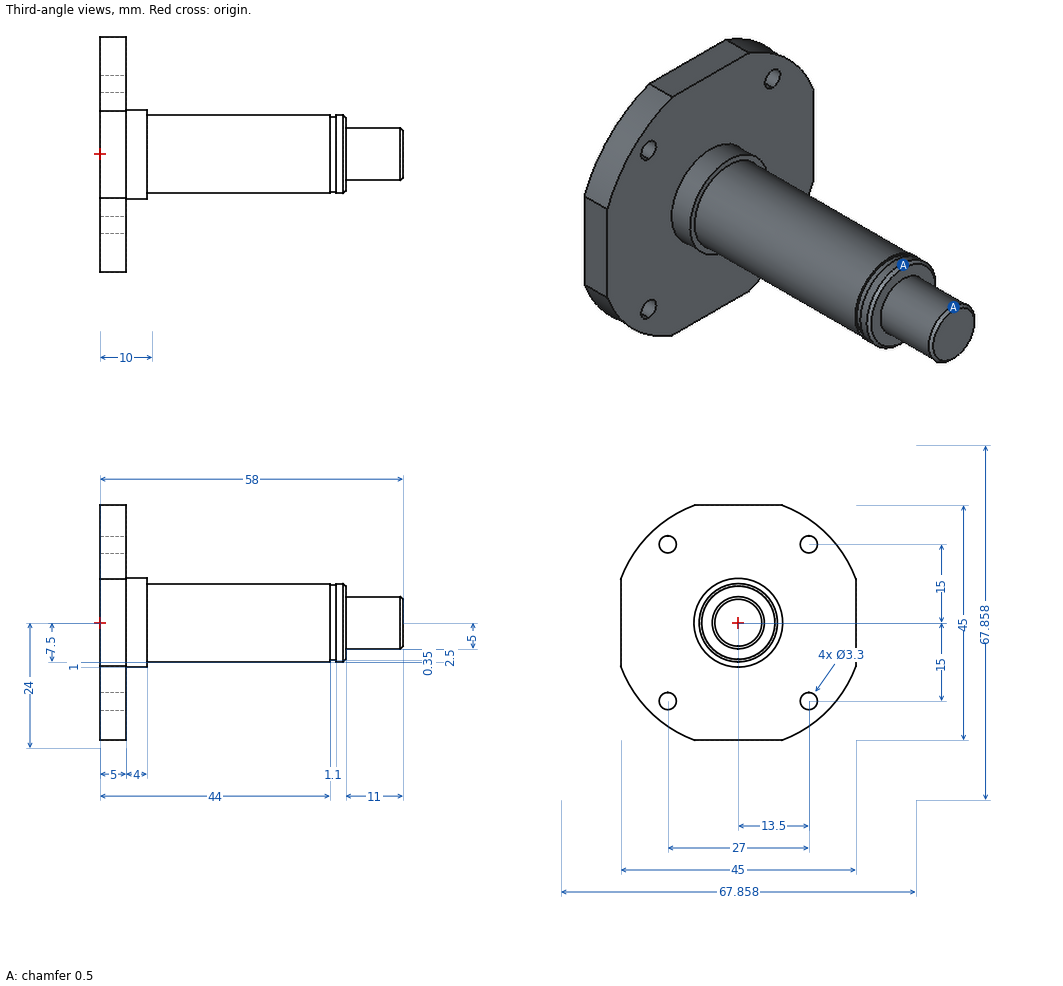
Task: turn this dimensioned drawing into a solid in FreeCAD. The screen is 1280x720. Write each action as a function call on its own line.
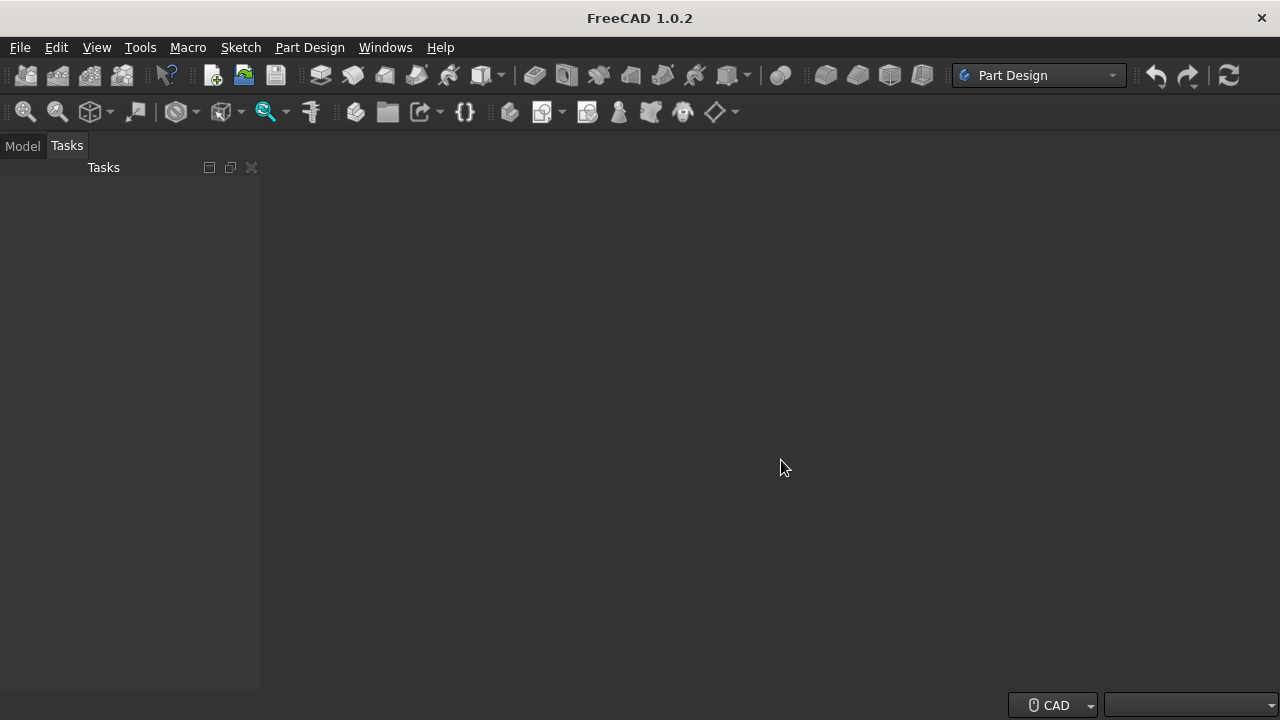
click(212, 76)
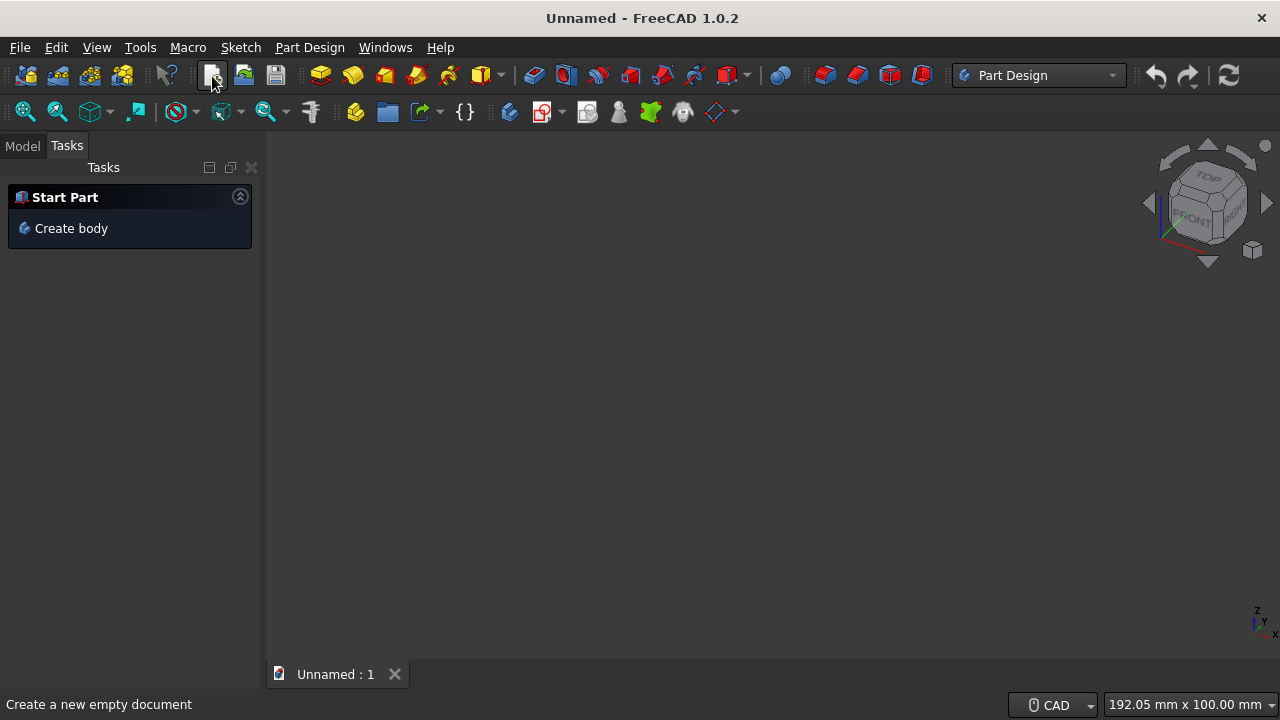
click(542, 112)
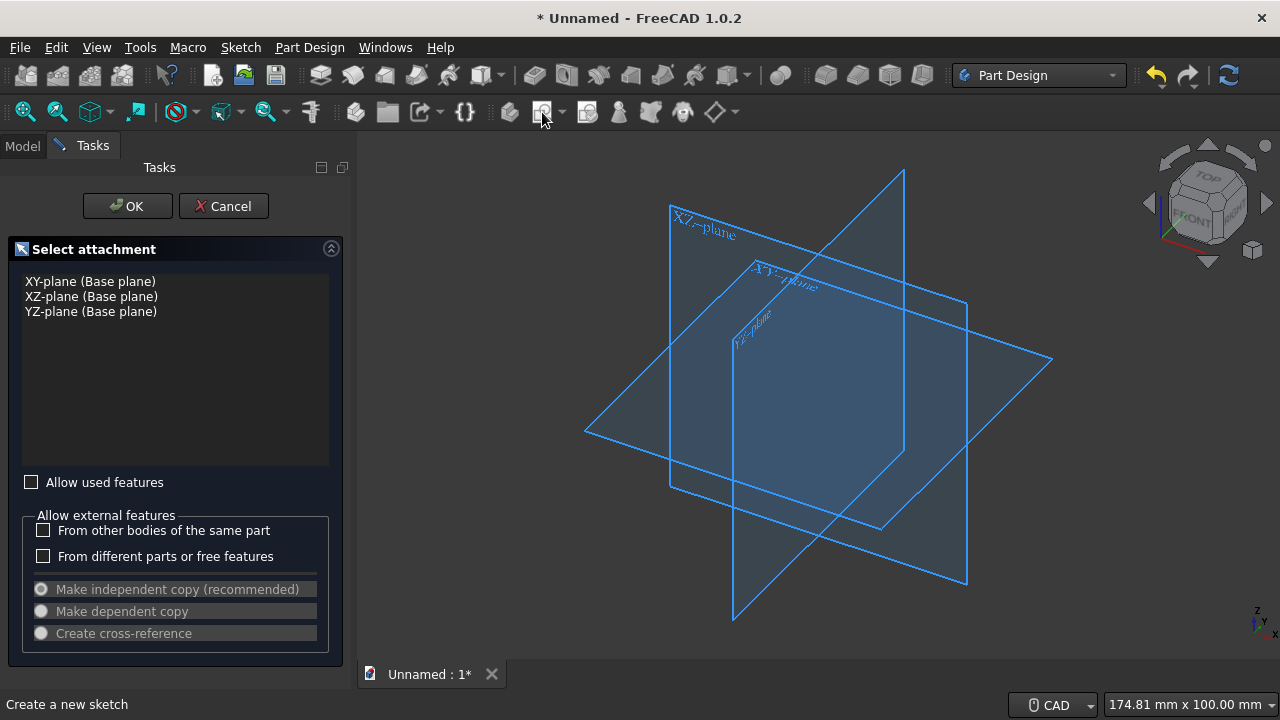
click(82, 296)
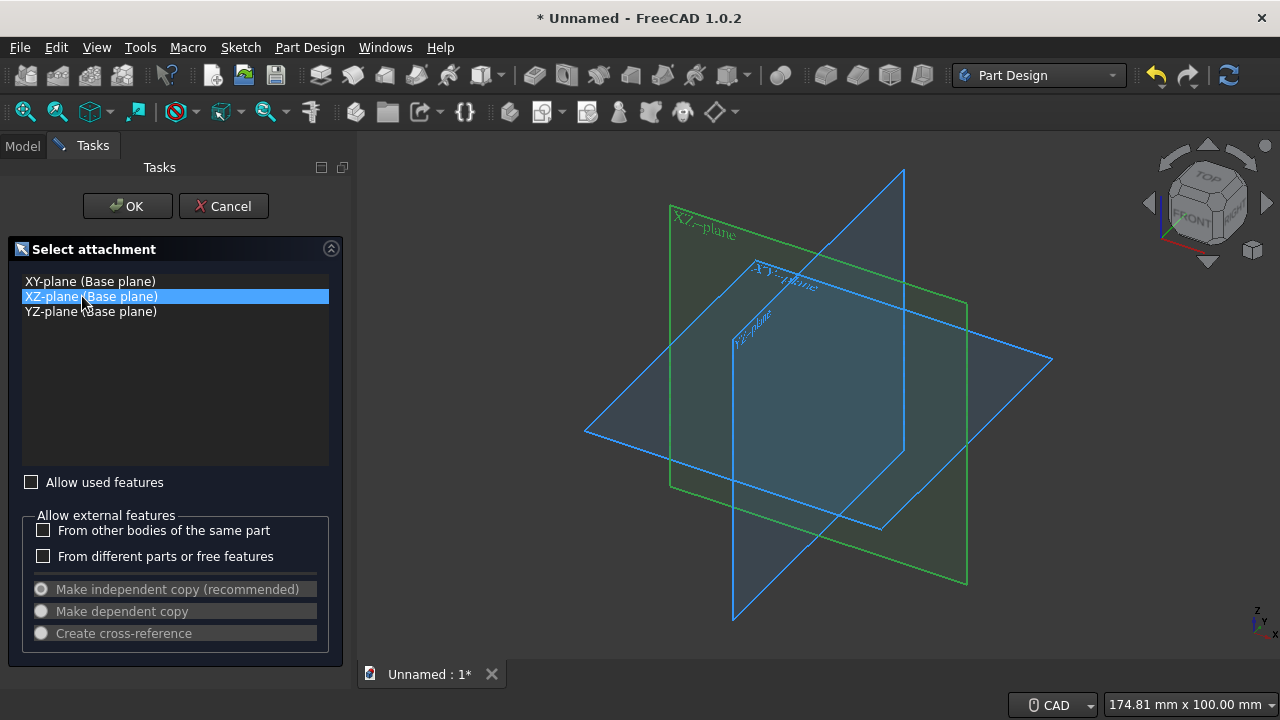
click(128, 206)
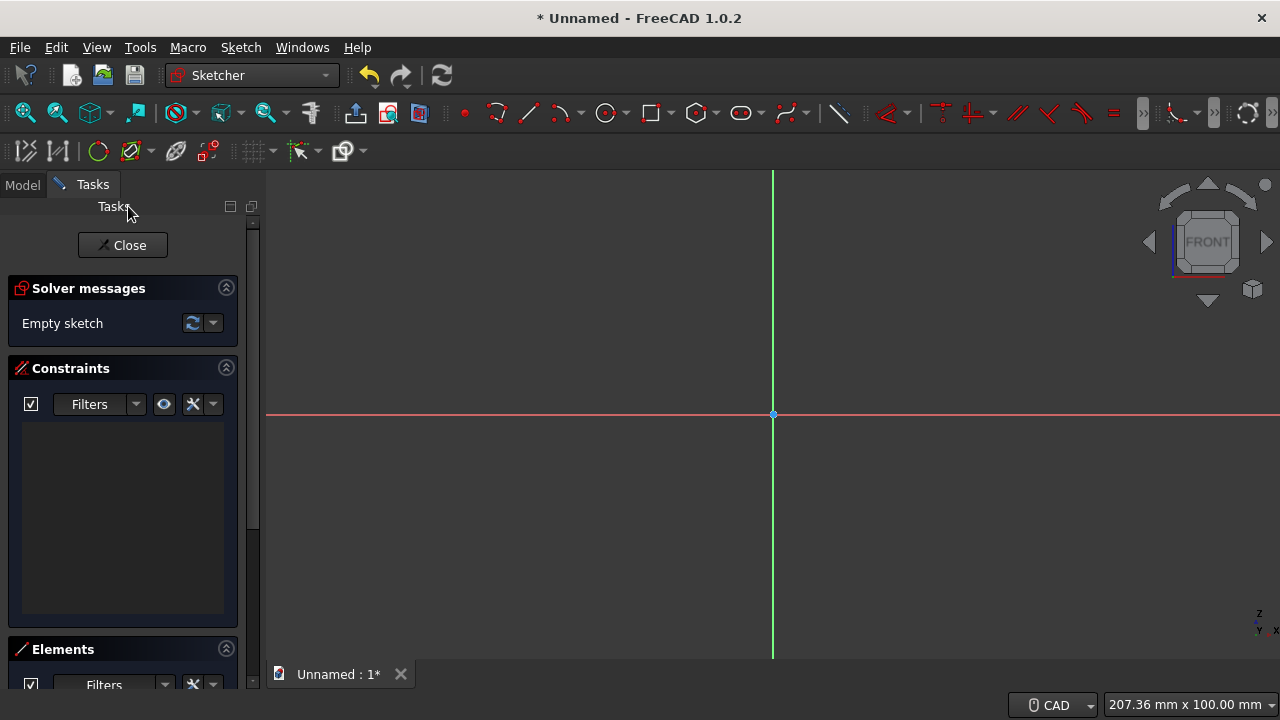
scroll(1086, 521, up, 4)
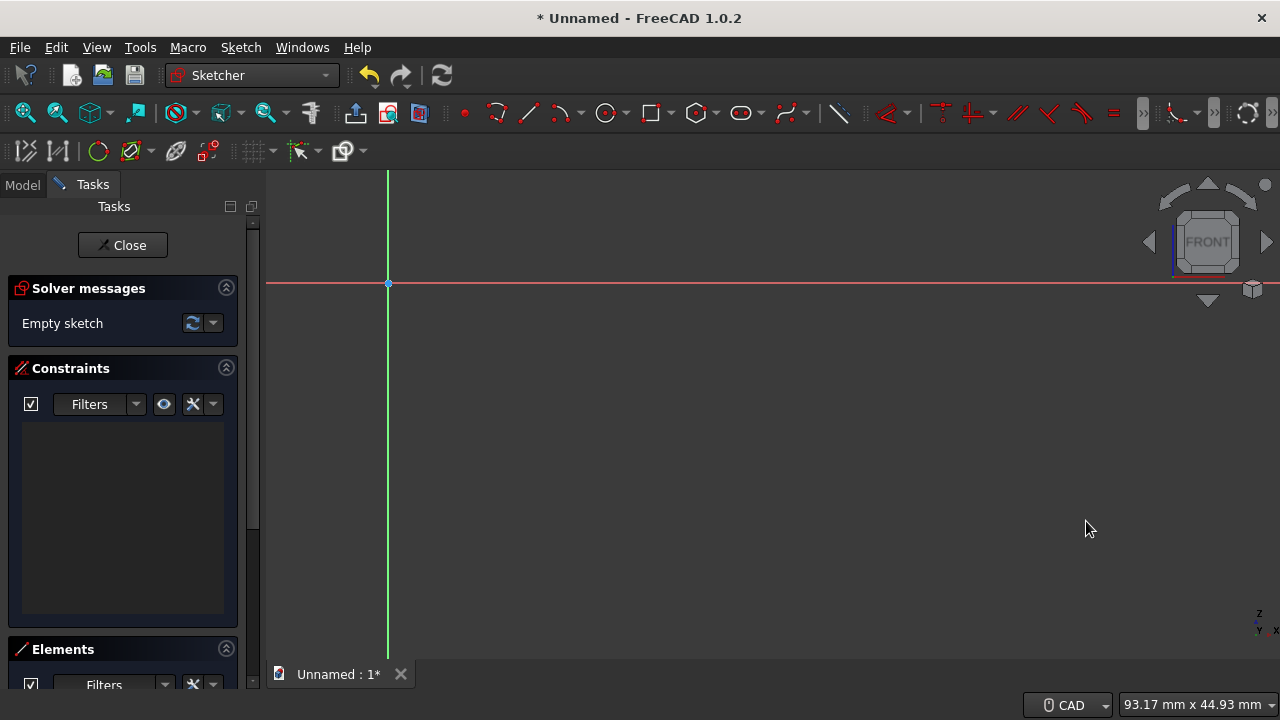
click(498, 114)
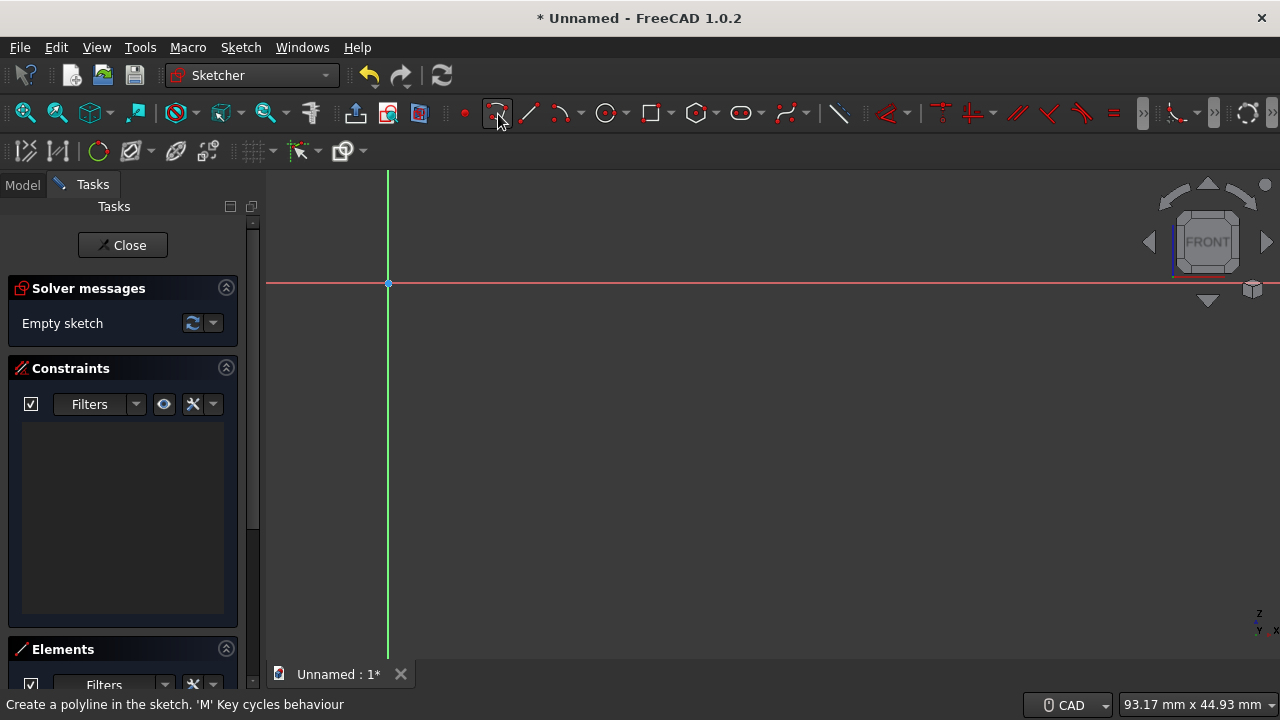
click(388, 283)
click(1020, 292)
click(1020, 338)
click(900, 338)
click(900, 365)
click(486, 365)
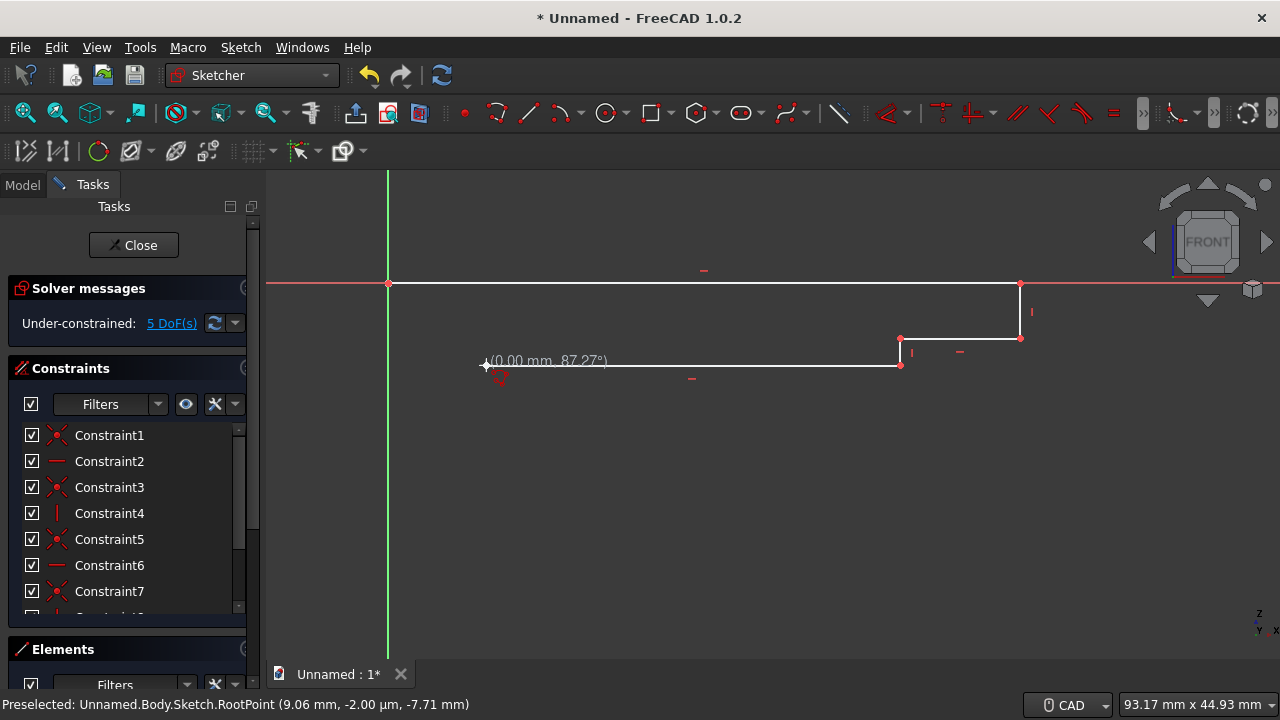
scroll(486, 376, up, 2)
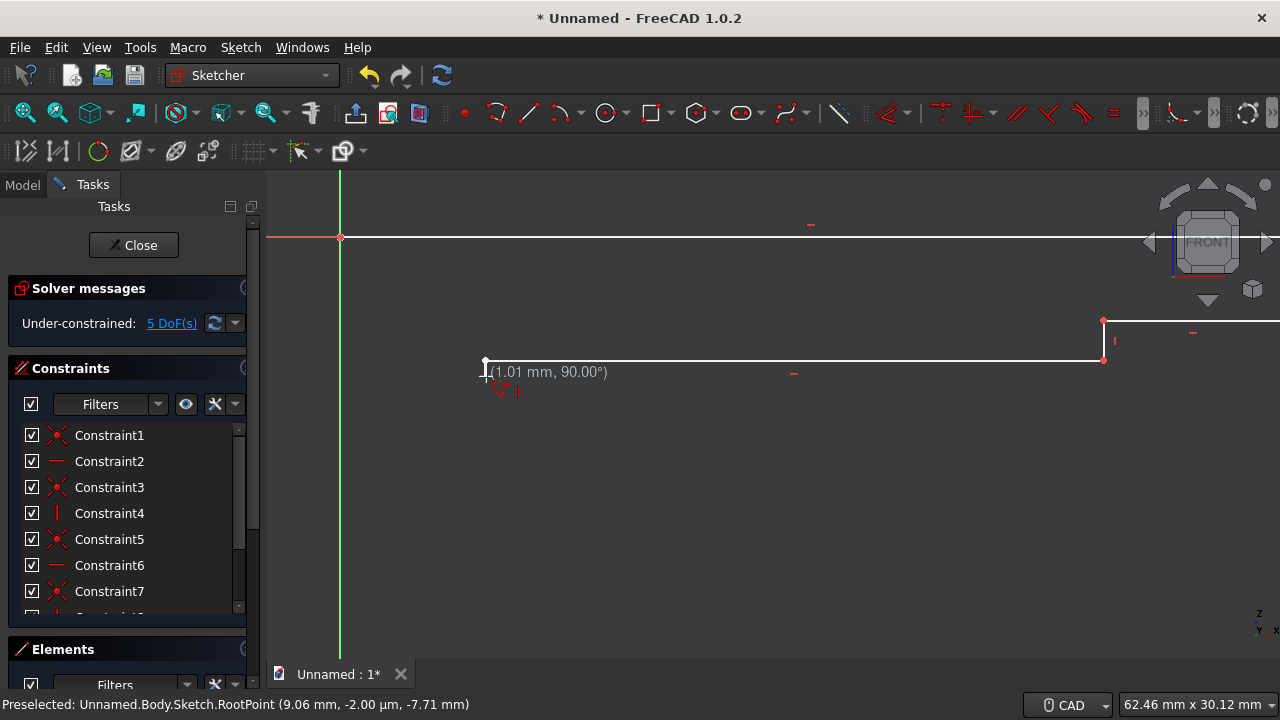
click(486, 375)
click(421, 375)
click(421, 627)
click(349, 627)
click(340, 237)
key(Escape)
key(Escape)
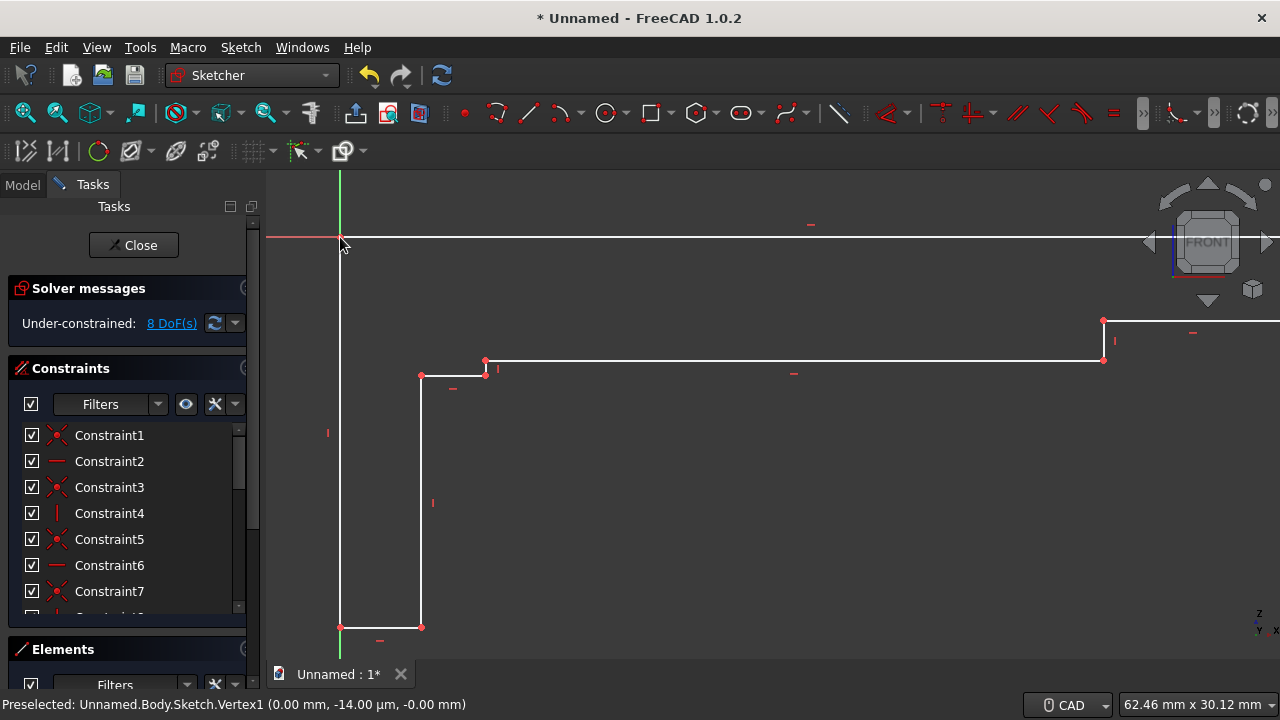
scroll(488, 379, down, 2)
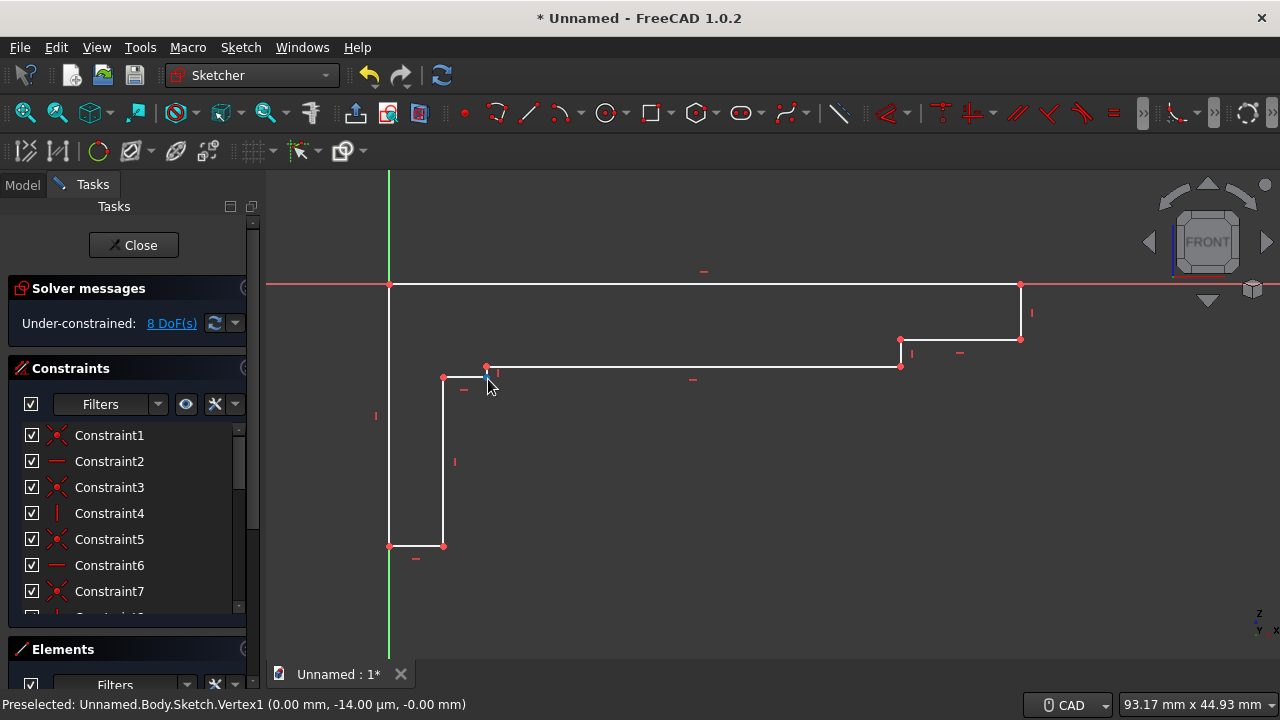
click(1021, 301)